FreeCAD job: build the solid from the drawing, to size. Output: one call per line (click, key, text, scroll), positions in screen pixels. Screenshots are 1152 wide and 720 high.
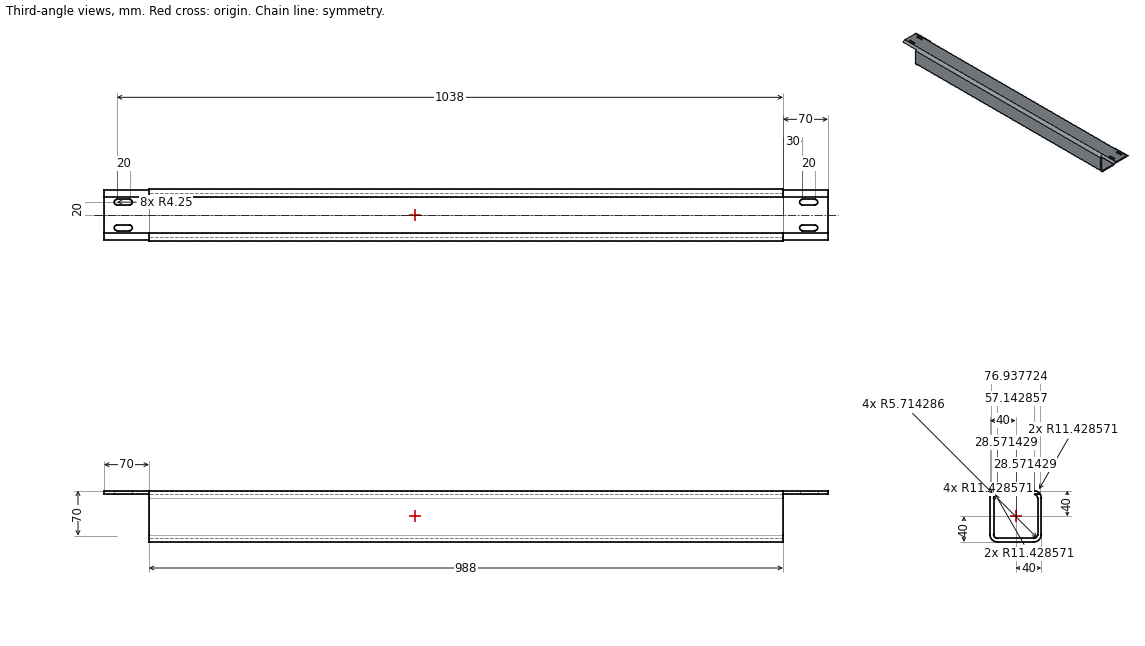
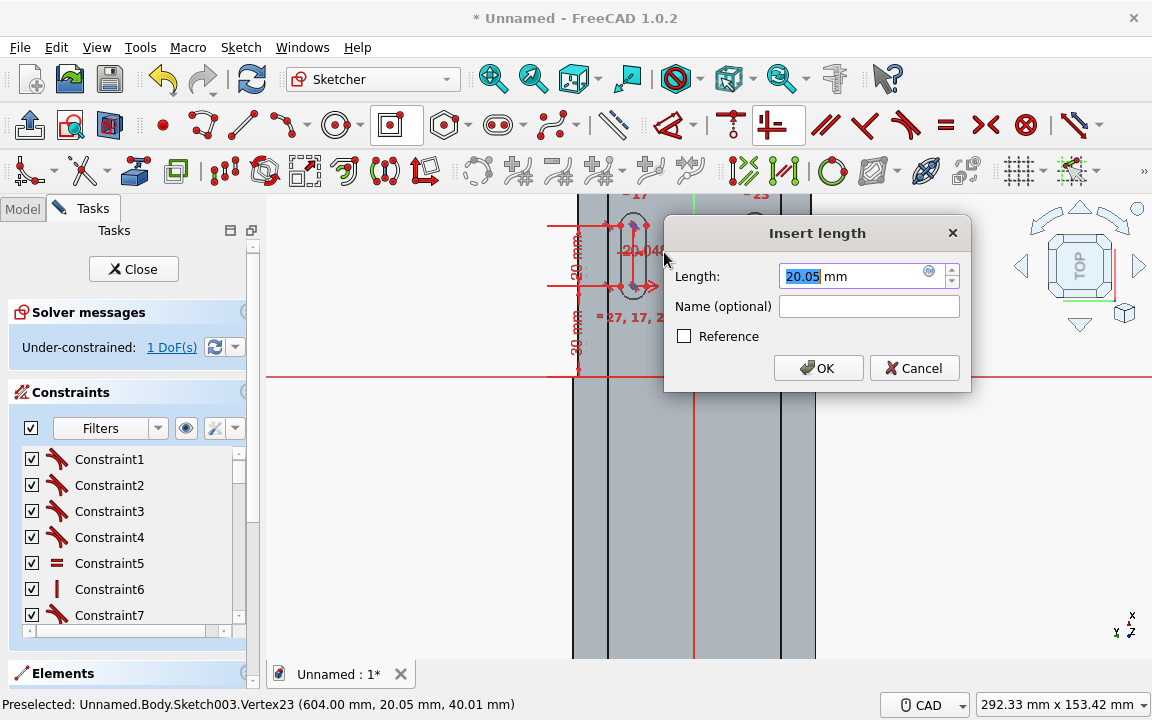
text(20)
key(Return)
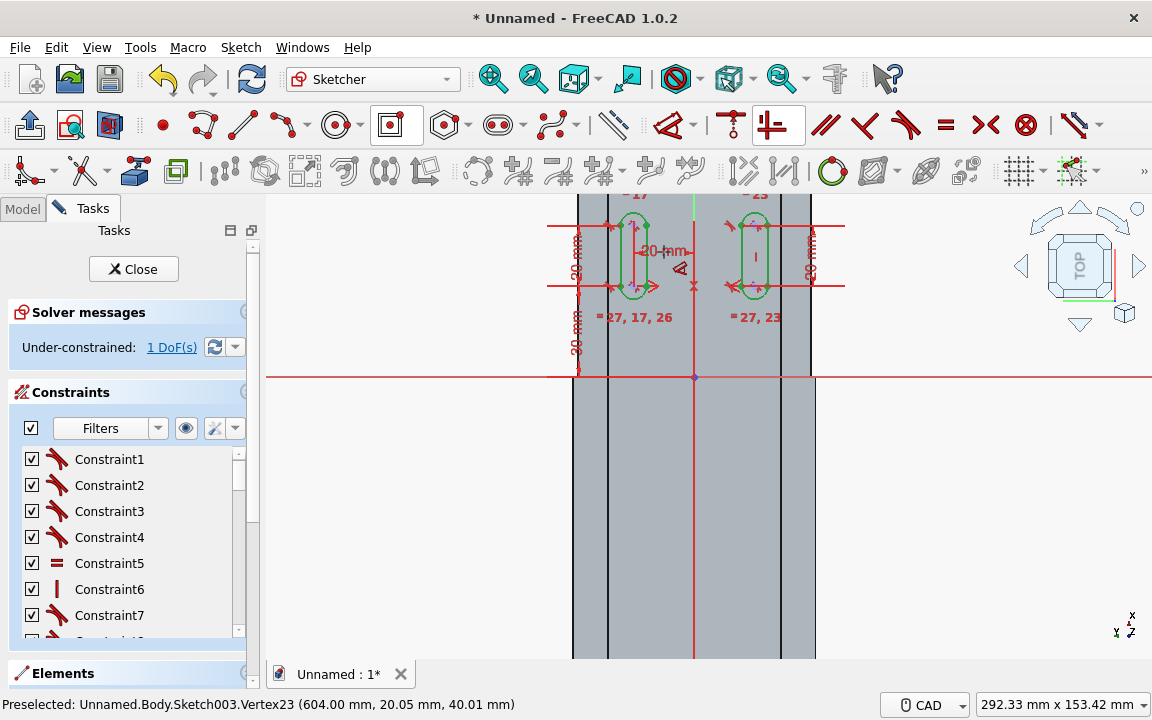
scroll(635, 282, down, 12)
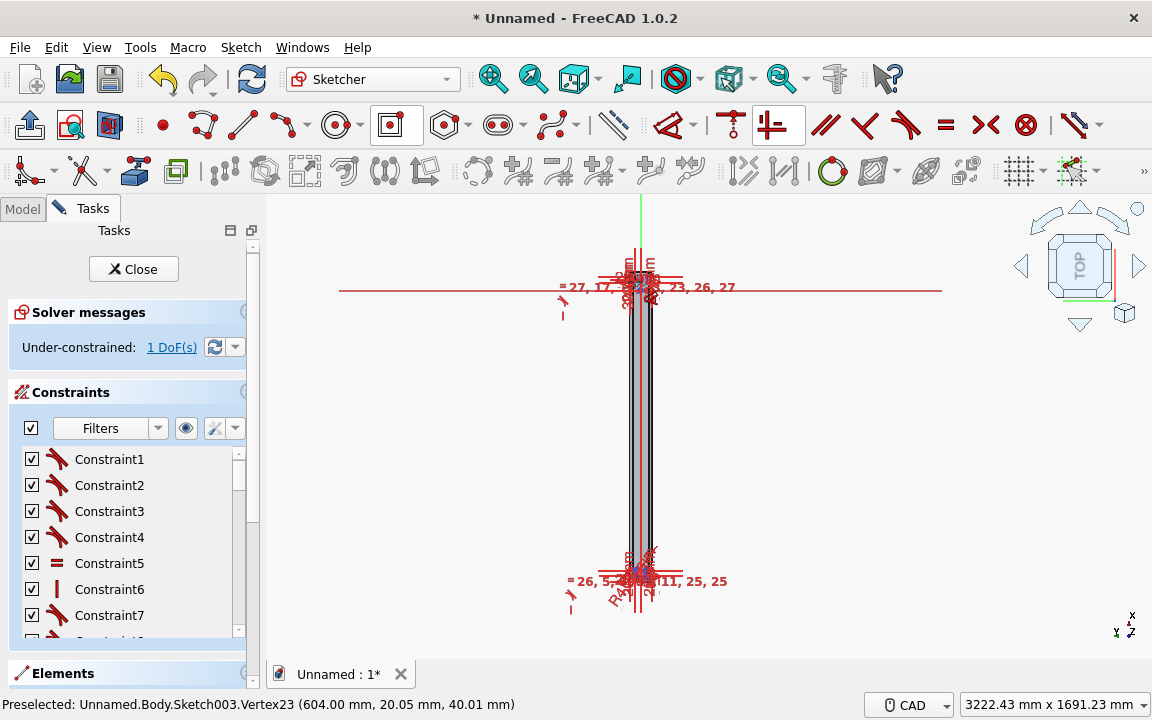
scroll(634, 576, up, 12)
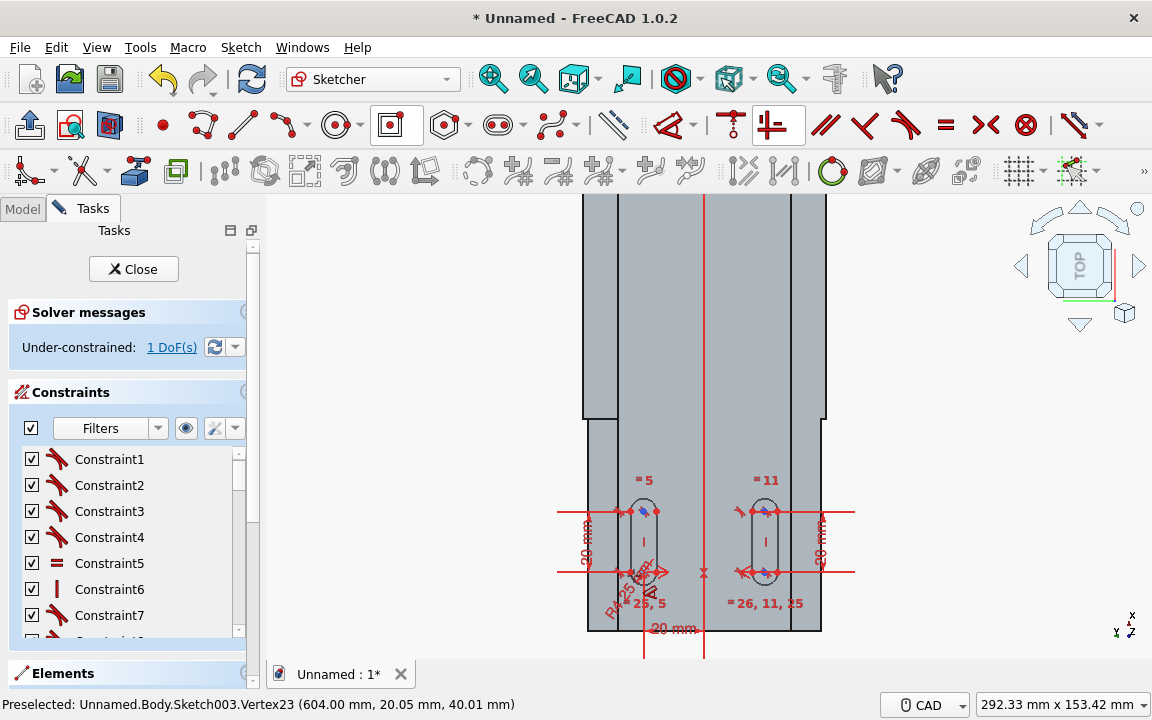
click(631, 572)
click(597, 397)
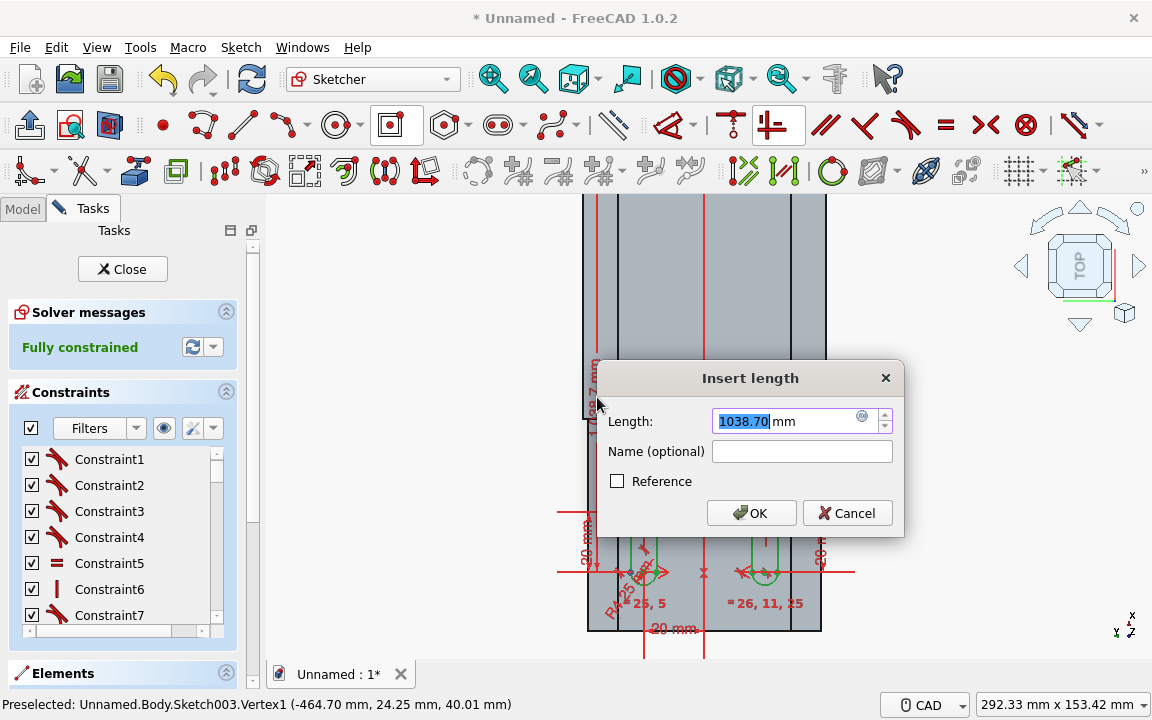
text(1038)
key(Return)
key(Escape)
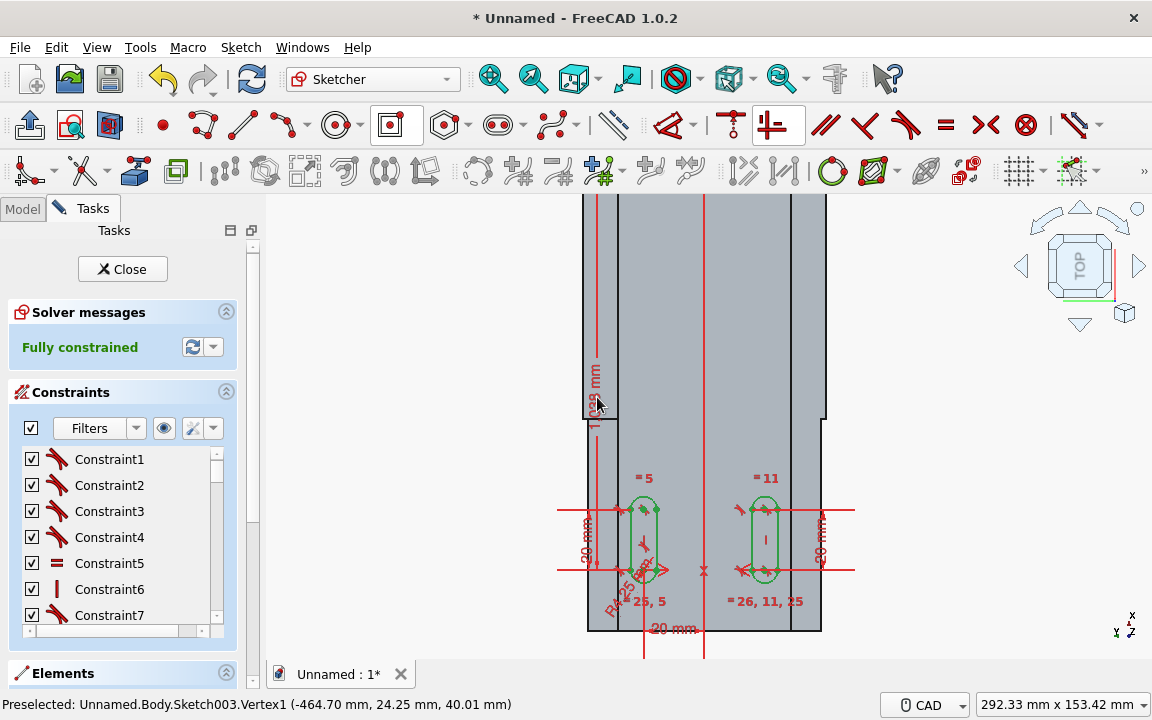
click(123, 269)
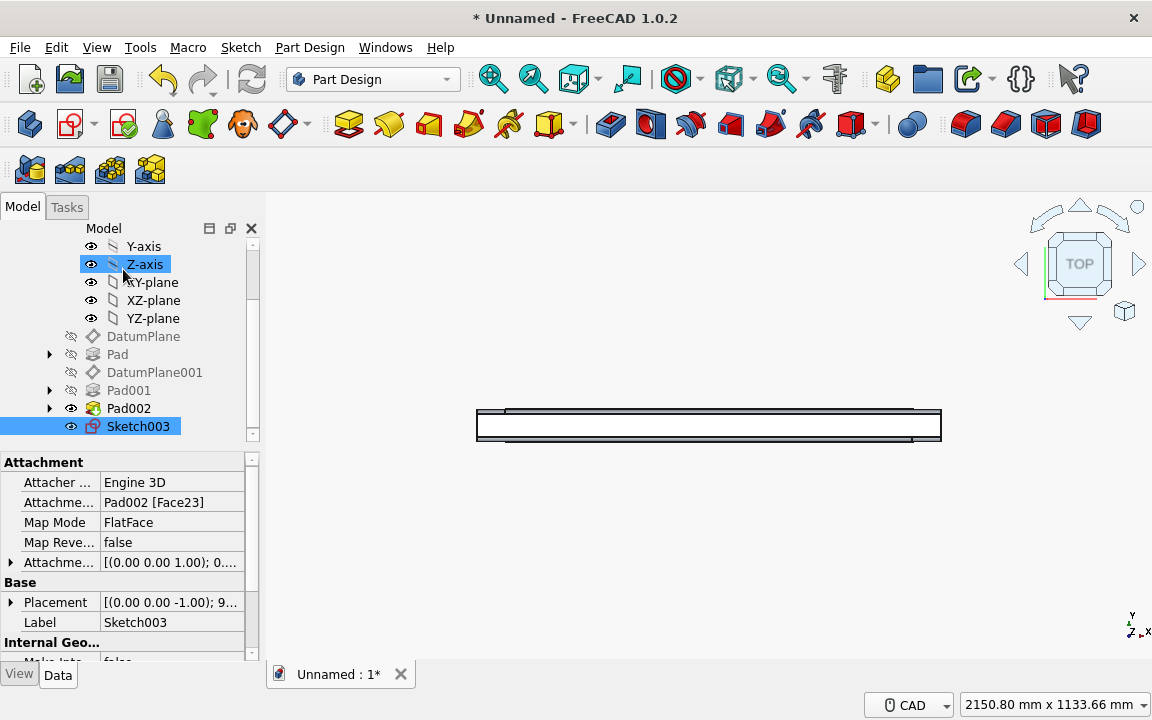
click(612, 124)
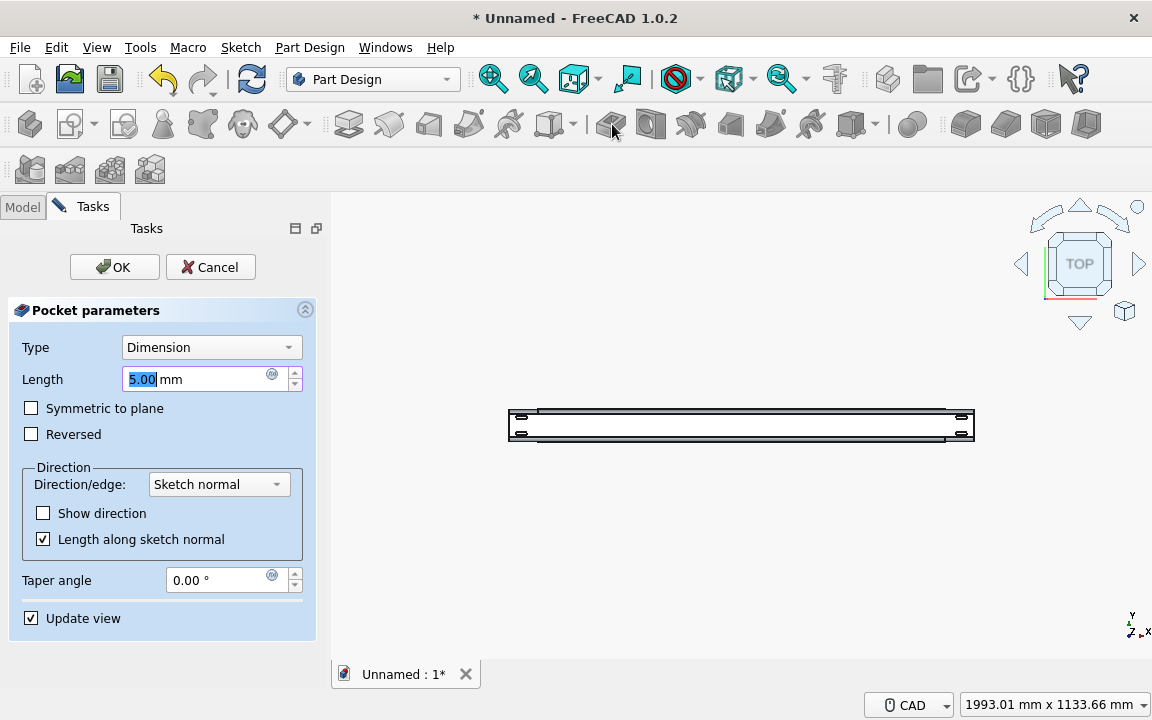
text(70)
key(Tab)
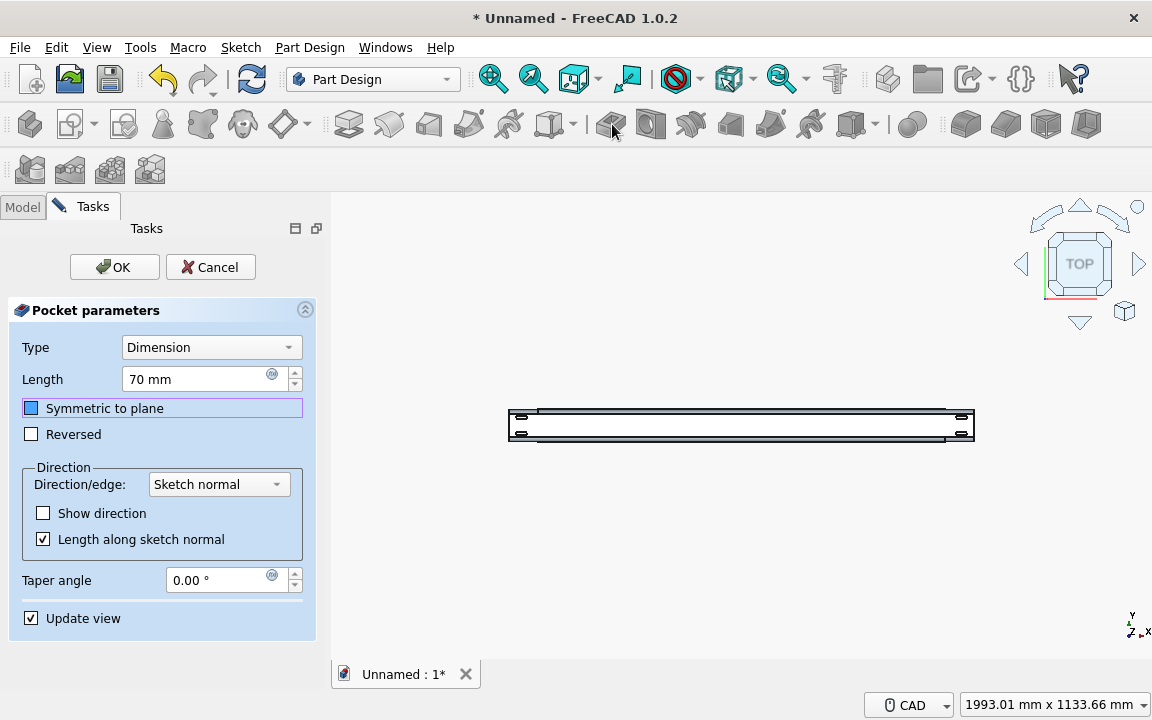
click(115, 267)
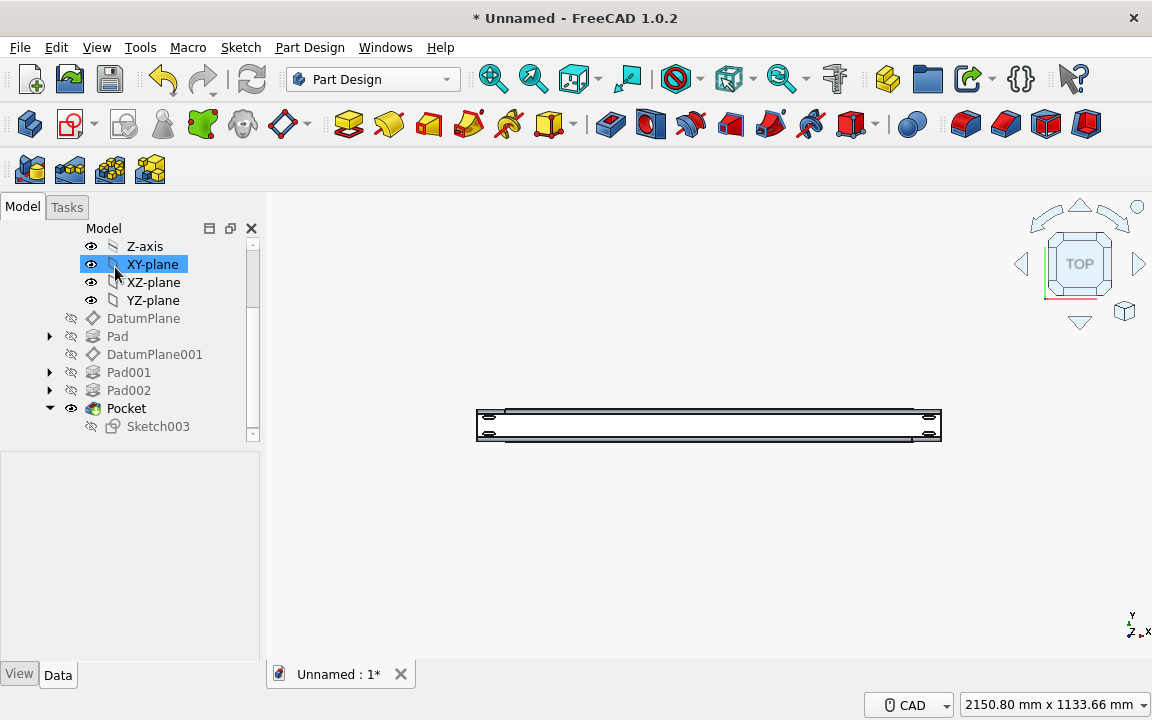
key(0)